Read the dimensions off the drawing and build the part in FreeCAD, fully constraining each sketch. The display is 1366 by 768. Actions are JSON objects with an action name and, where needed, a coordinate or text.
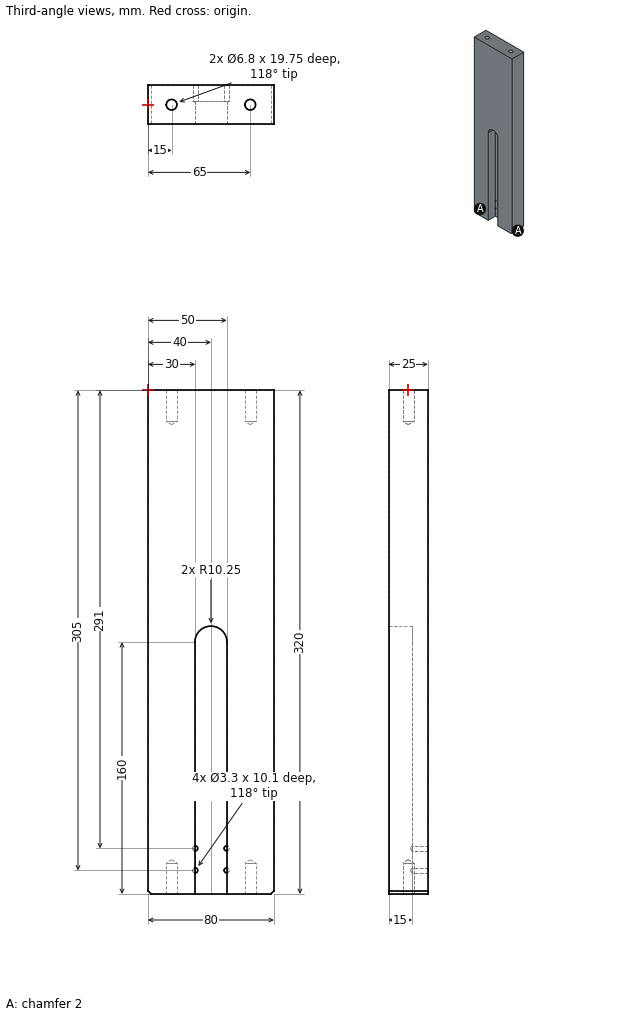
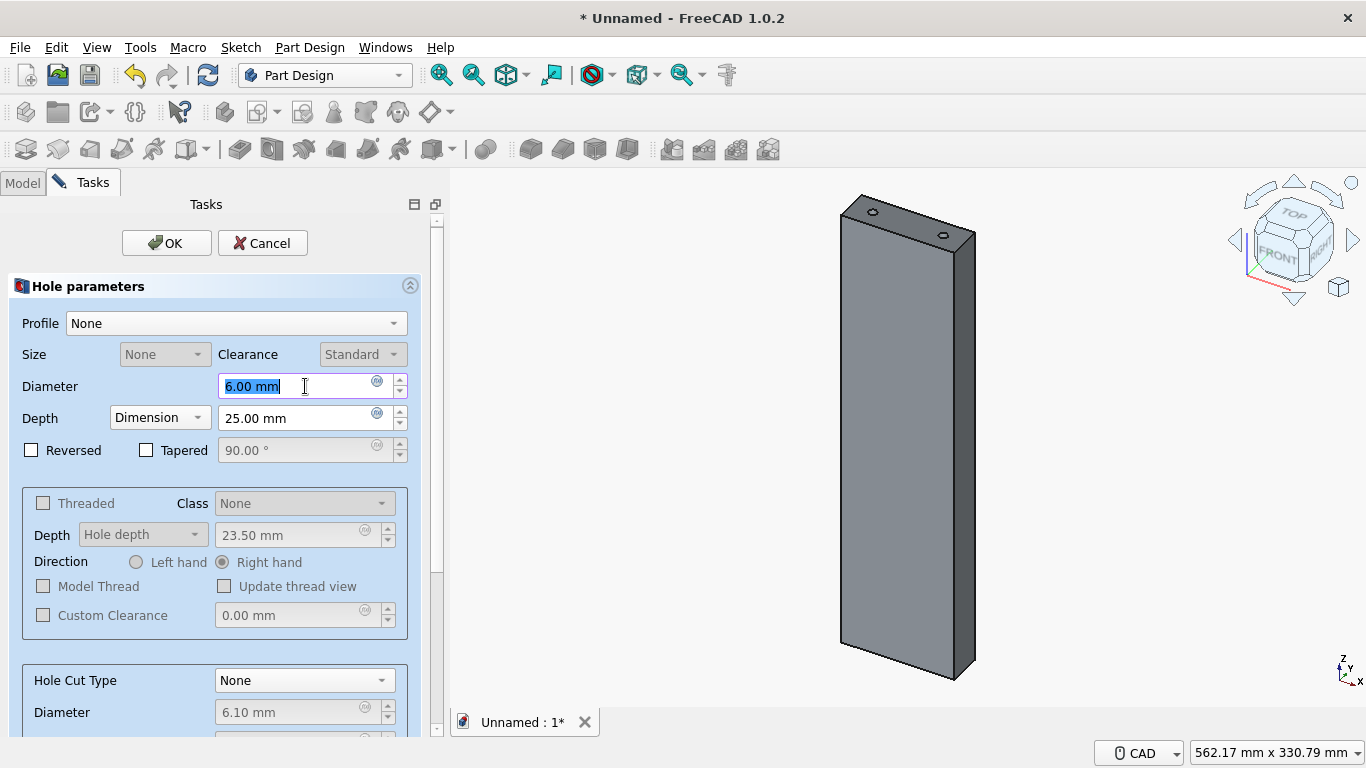
{"action": "type", "text": "6.8"}
{"action": "key", "text": "Tab"}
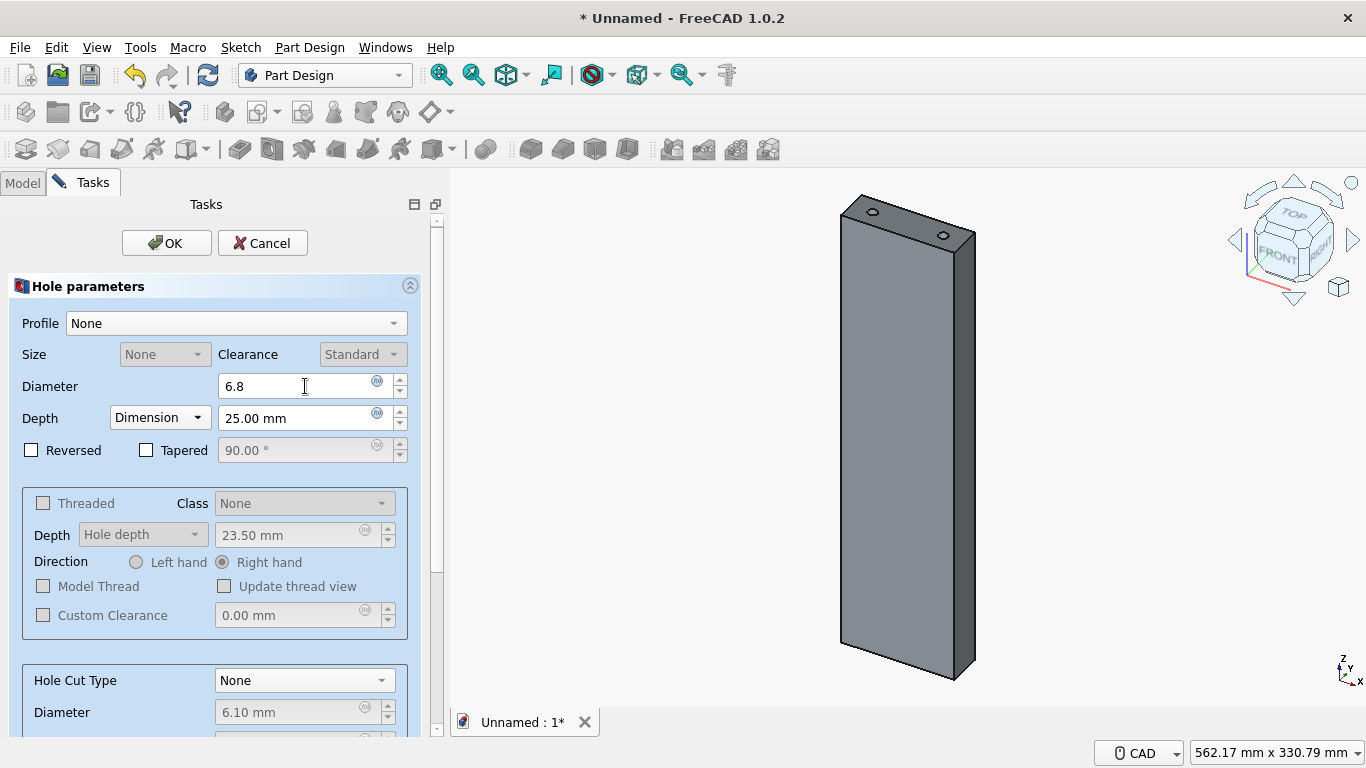
{"action": "triple_click", "coordinate": [305, 418]}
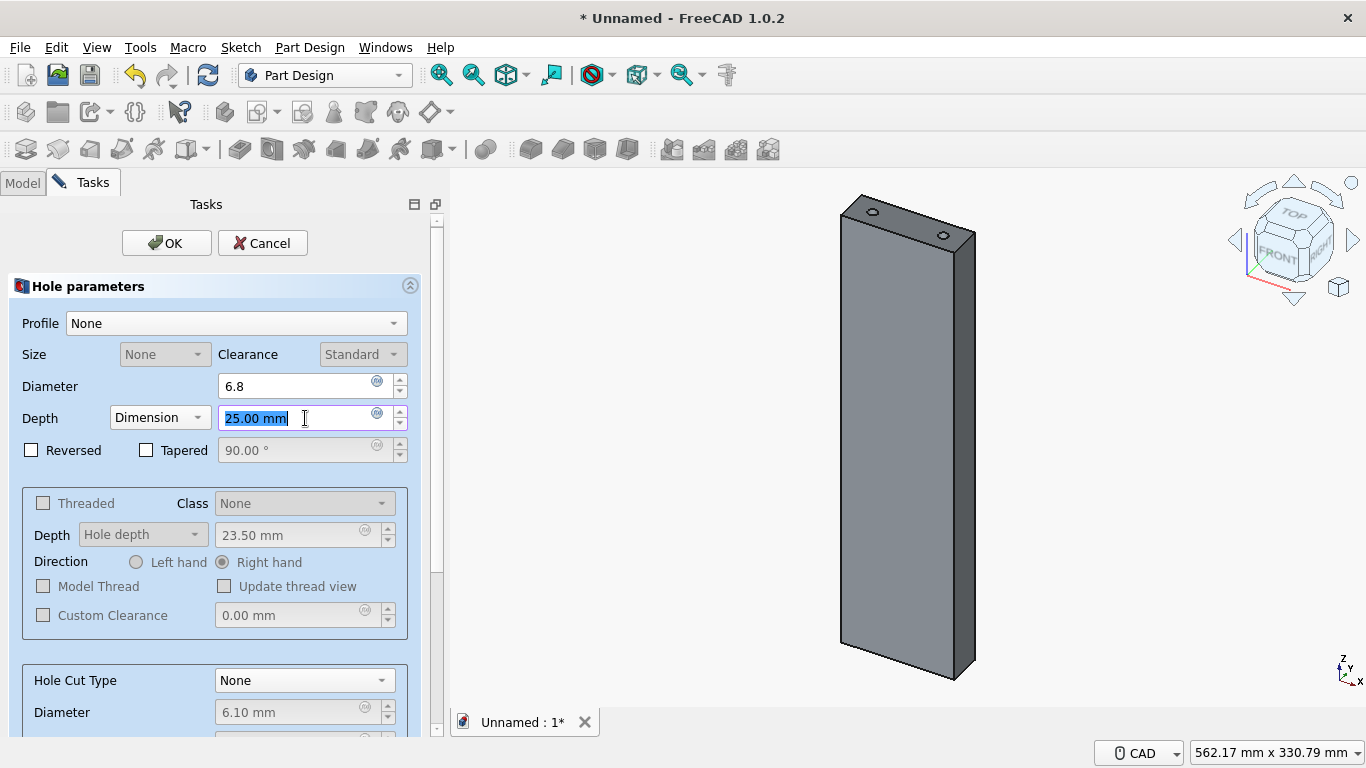
{"action": "type", "text": "19.75"}
{"action": "key", "text": "Tab"}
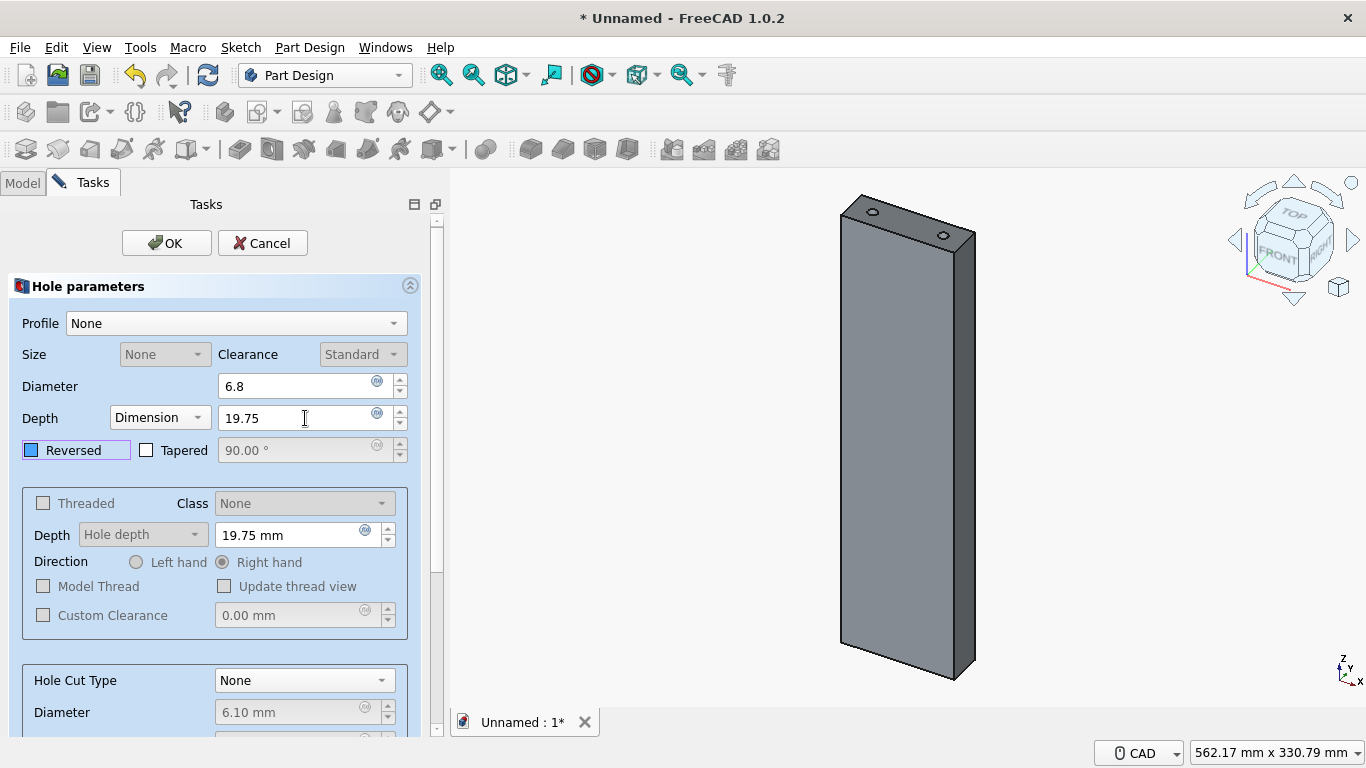
{"action": "left_click", "coordinate": [167, 243]}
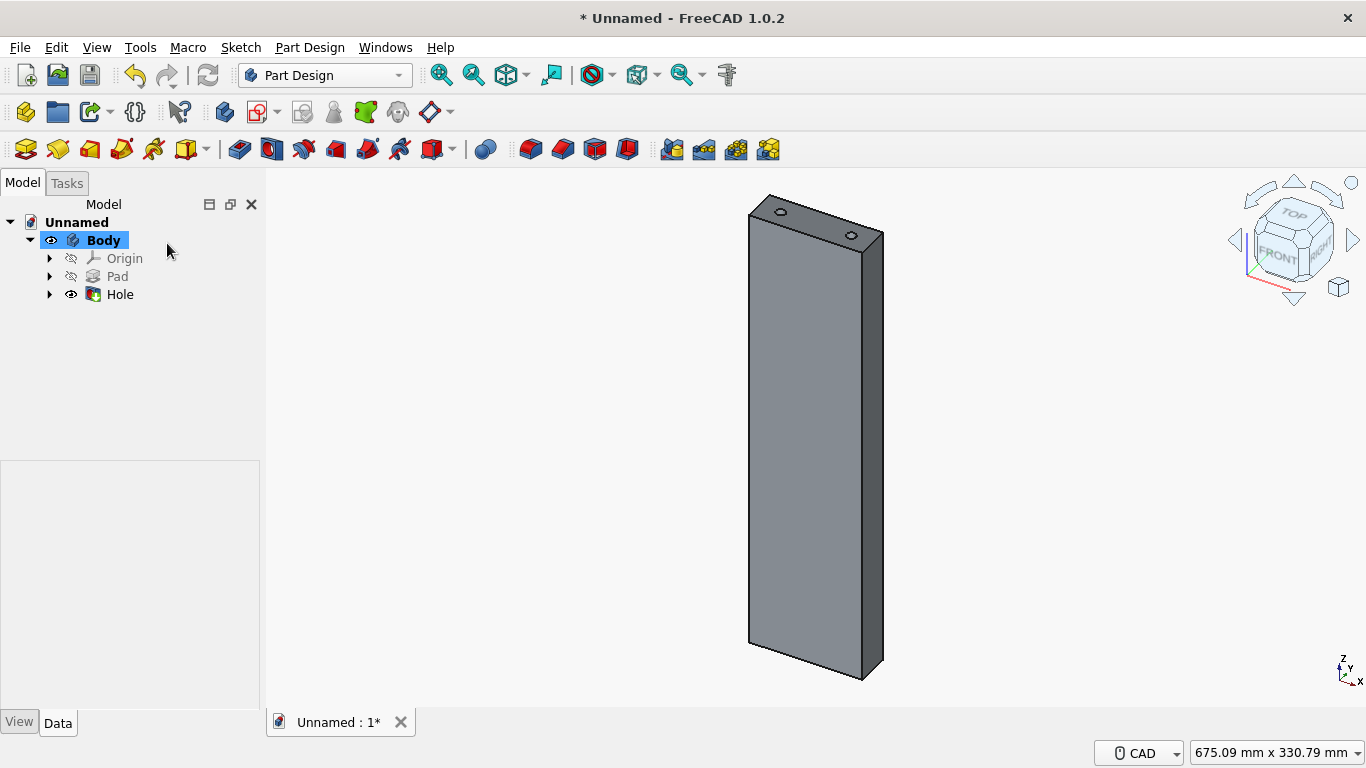
{"action": "key", "text": "0"}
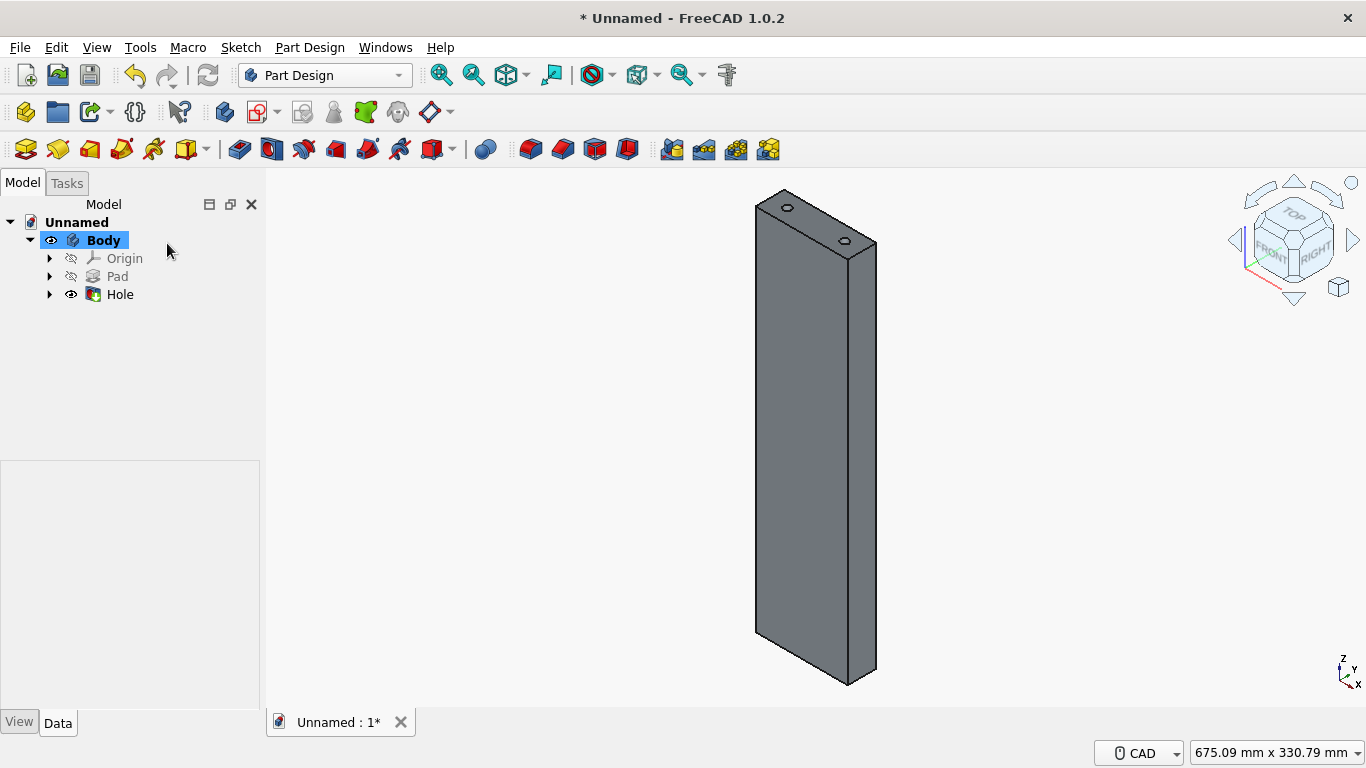
{"action": "key", "text": "2"}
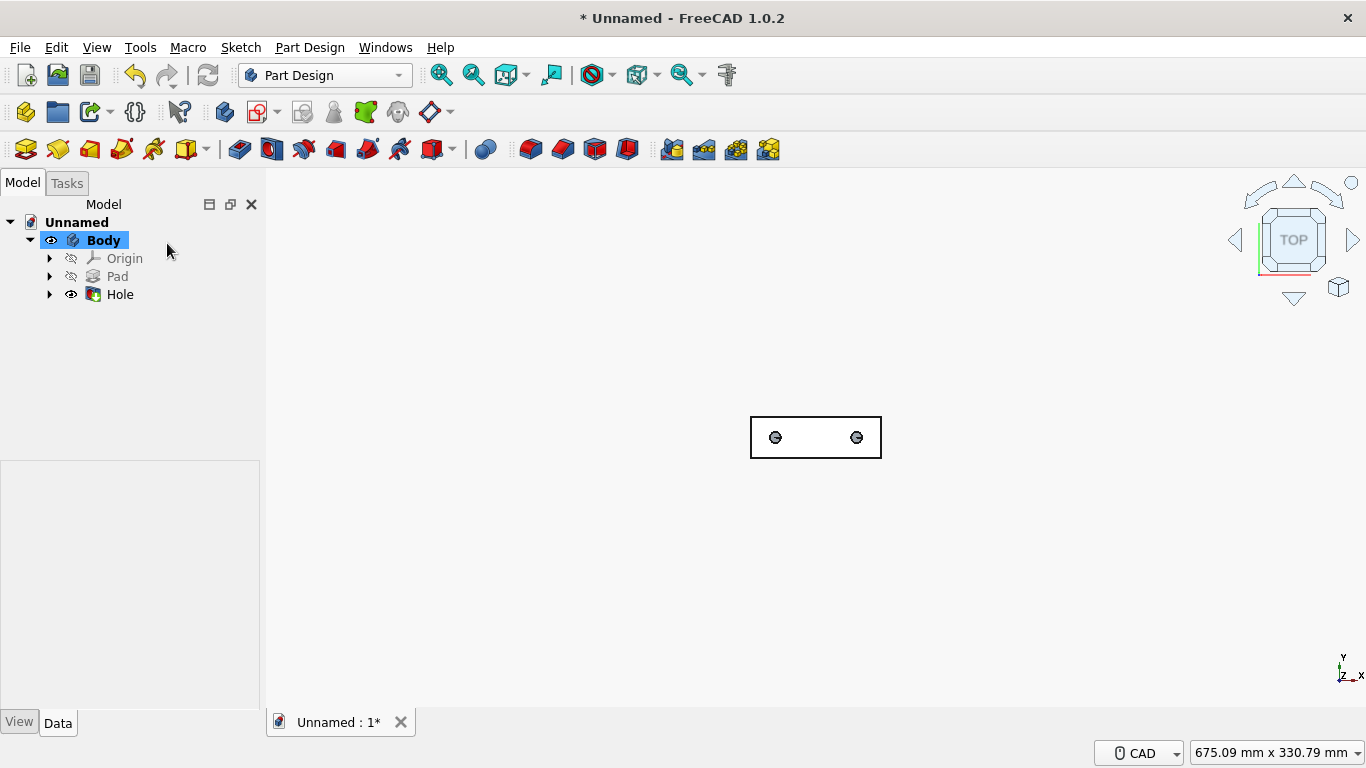
{"action": "left_click", "coordinate": [442, 76]}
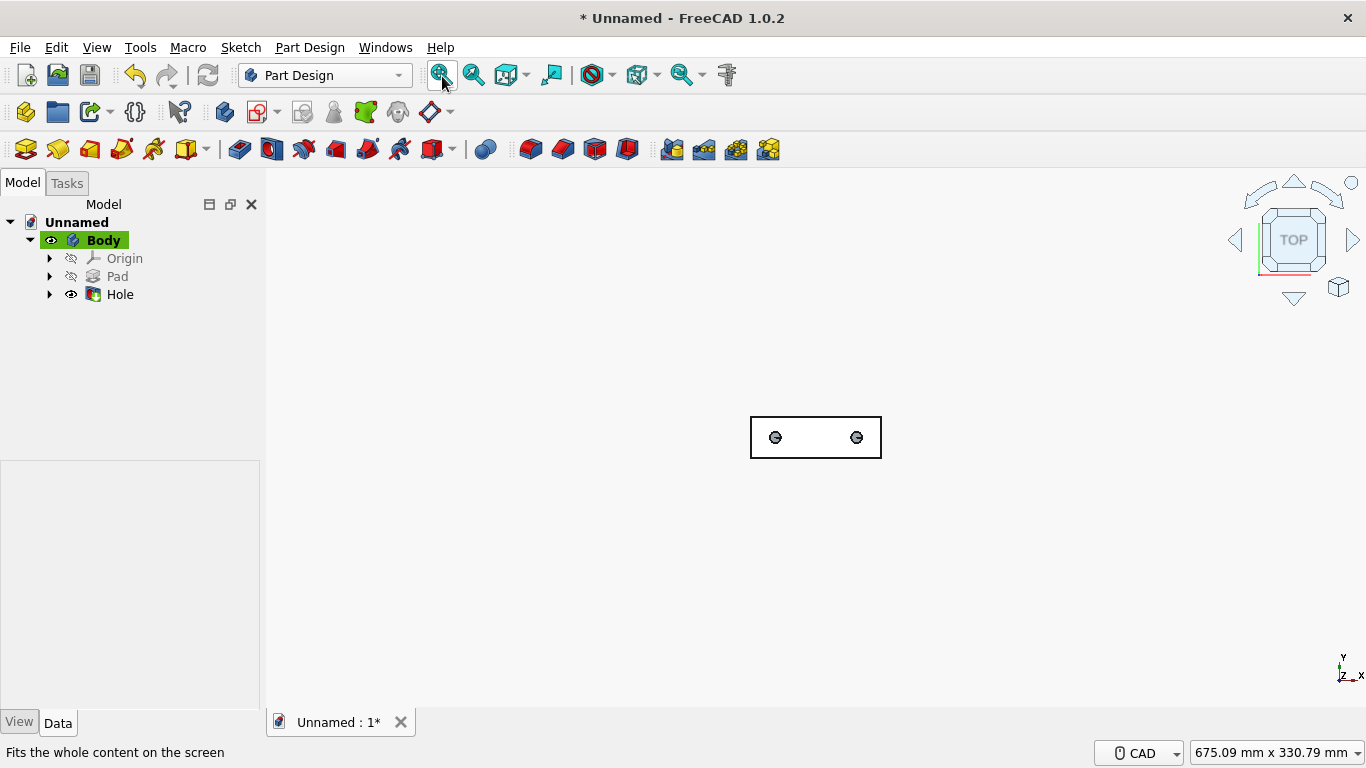
{"action": "key", "text": "1"}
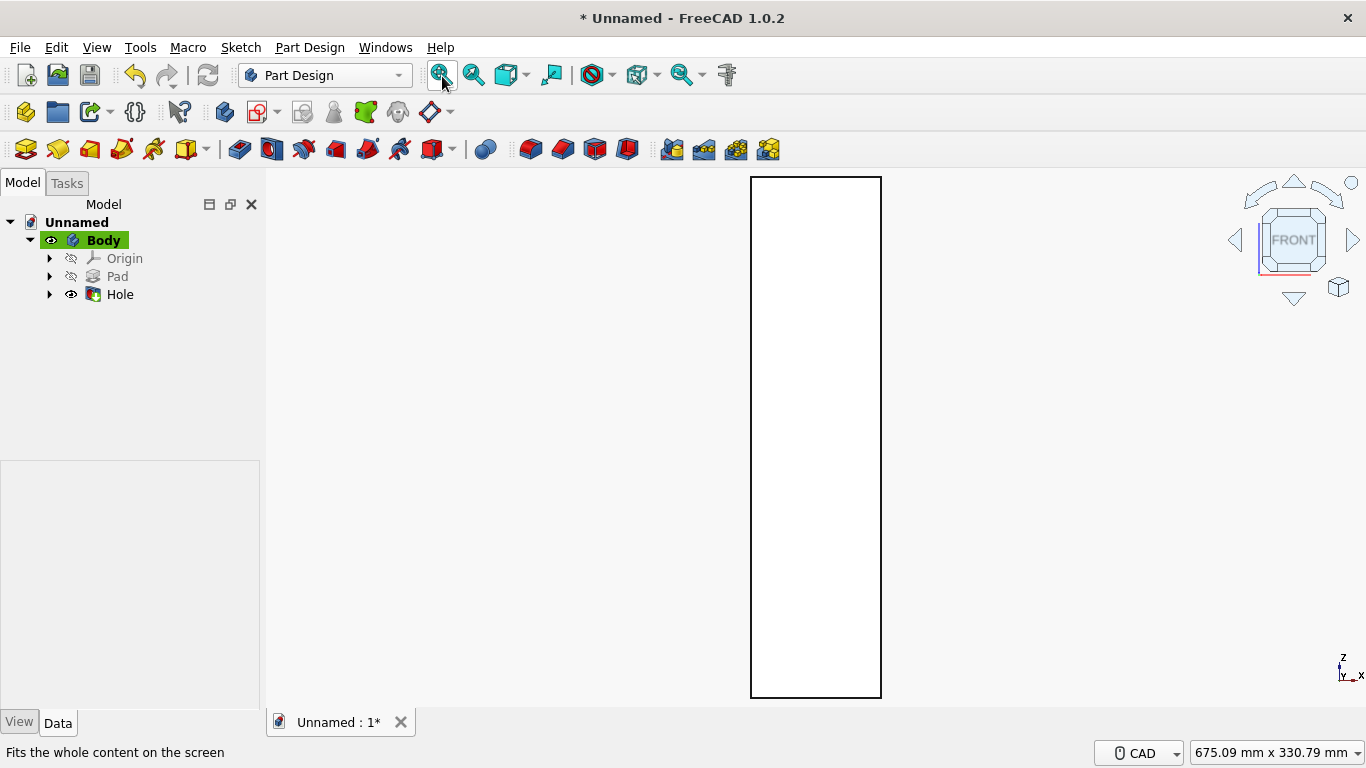
{"action": "key", "text": "3"}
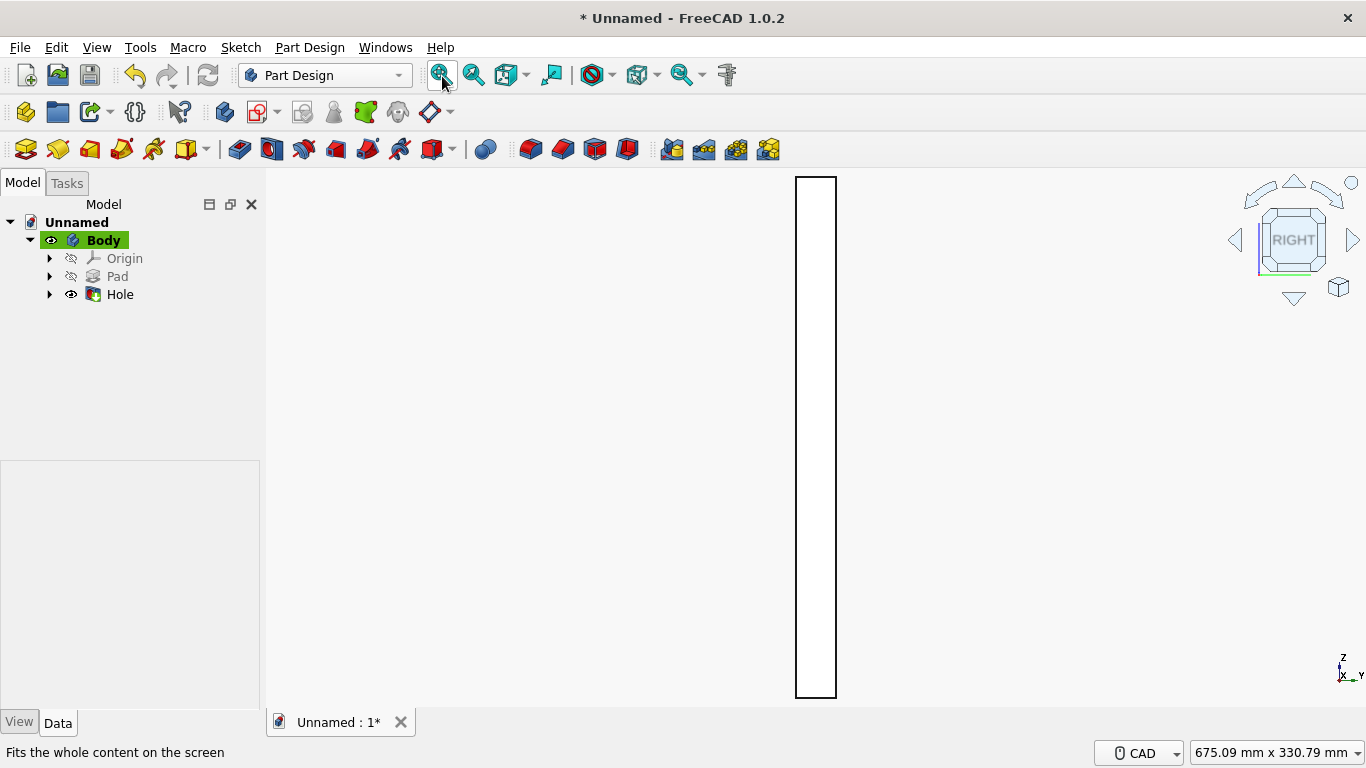
{"action": "key", "text": "5"}